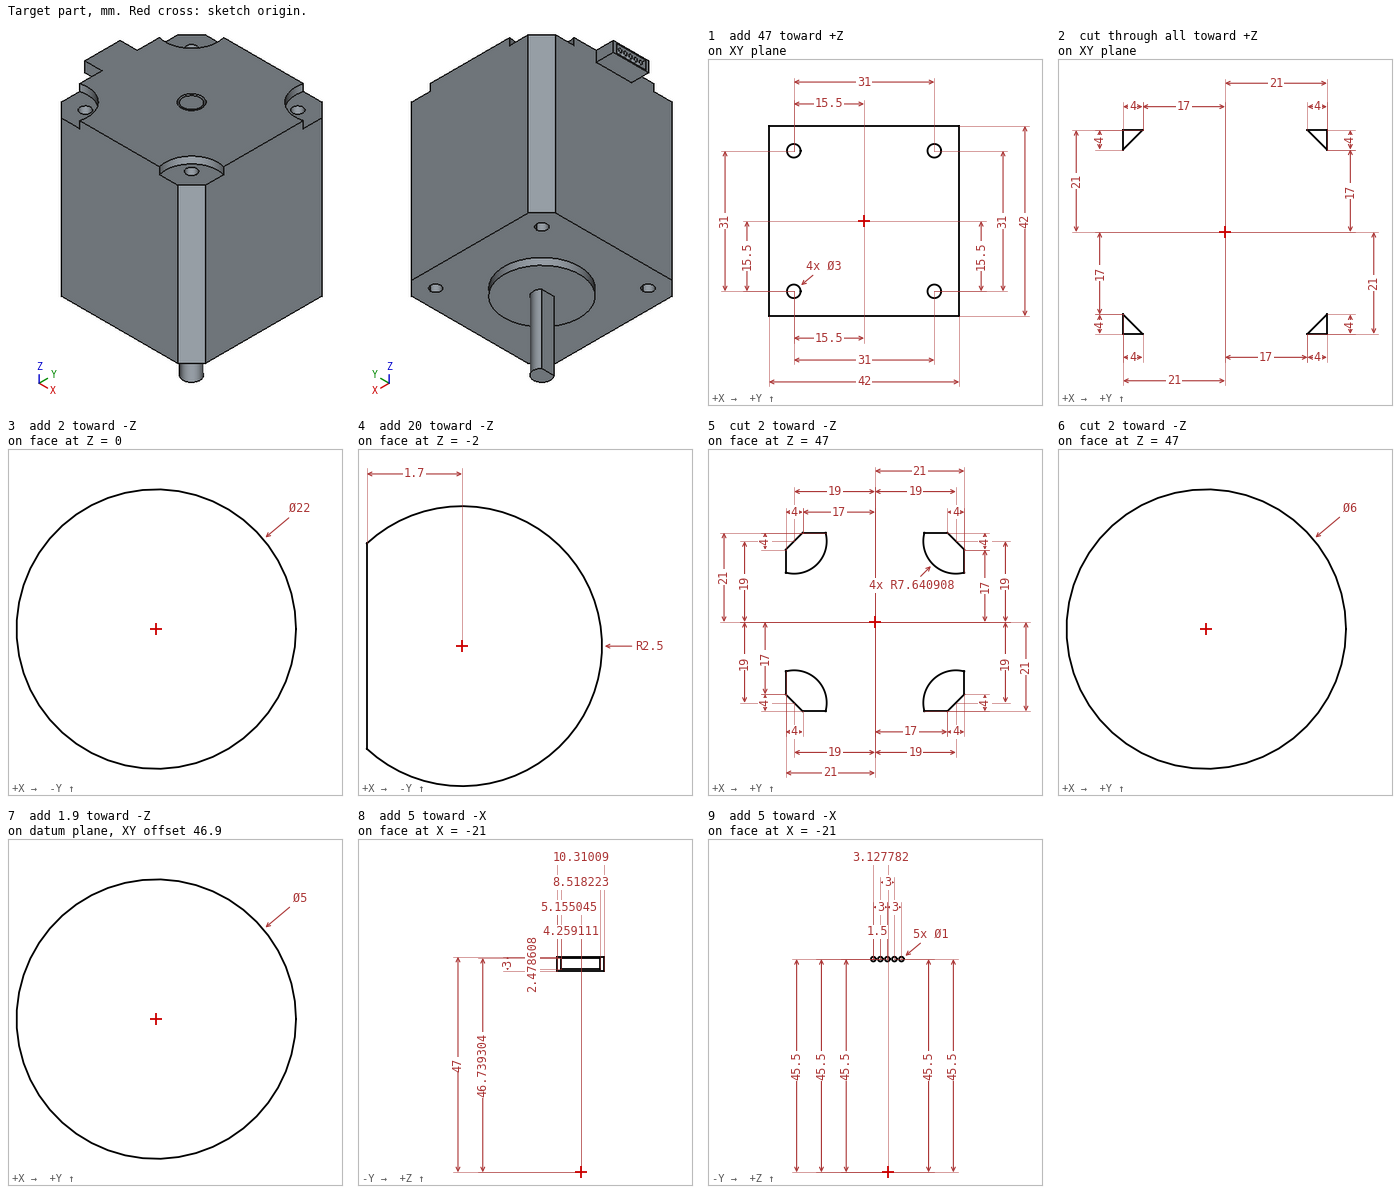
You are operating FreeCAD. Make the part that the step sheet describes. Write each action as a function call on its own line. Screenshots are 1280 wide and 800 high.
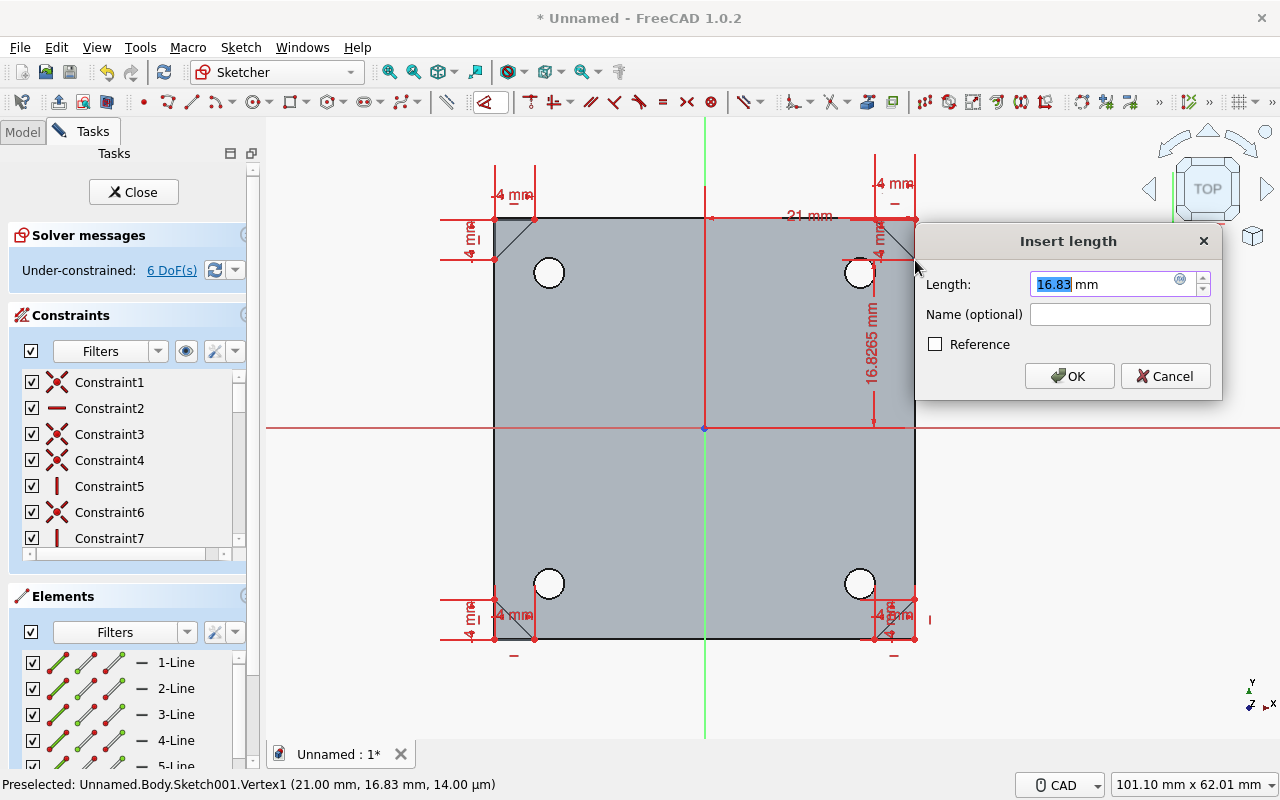
text(17)
key(Return)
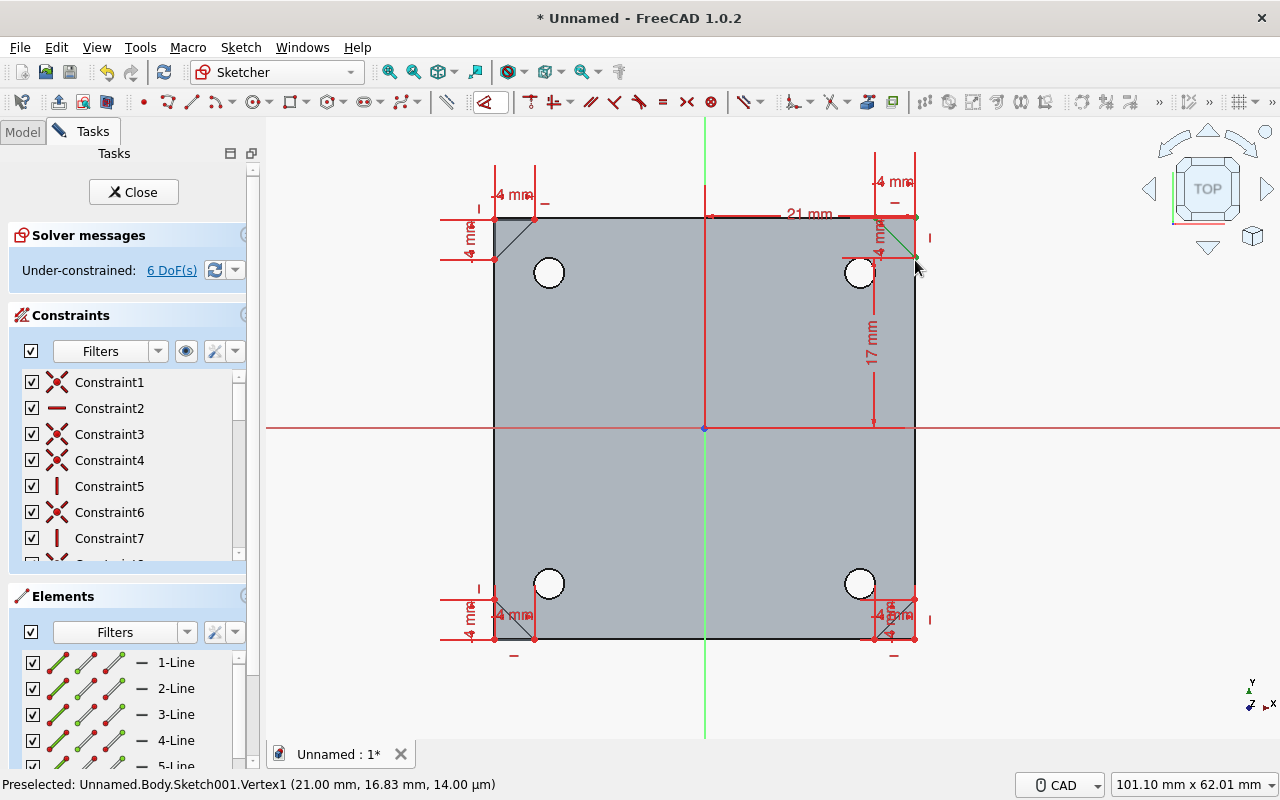
click(535, 220)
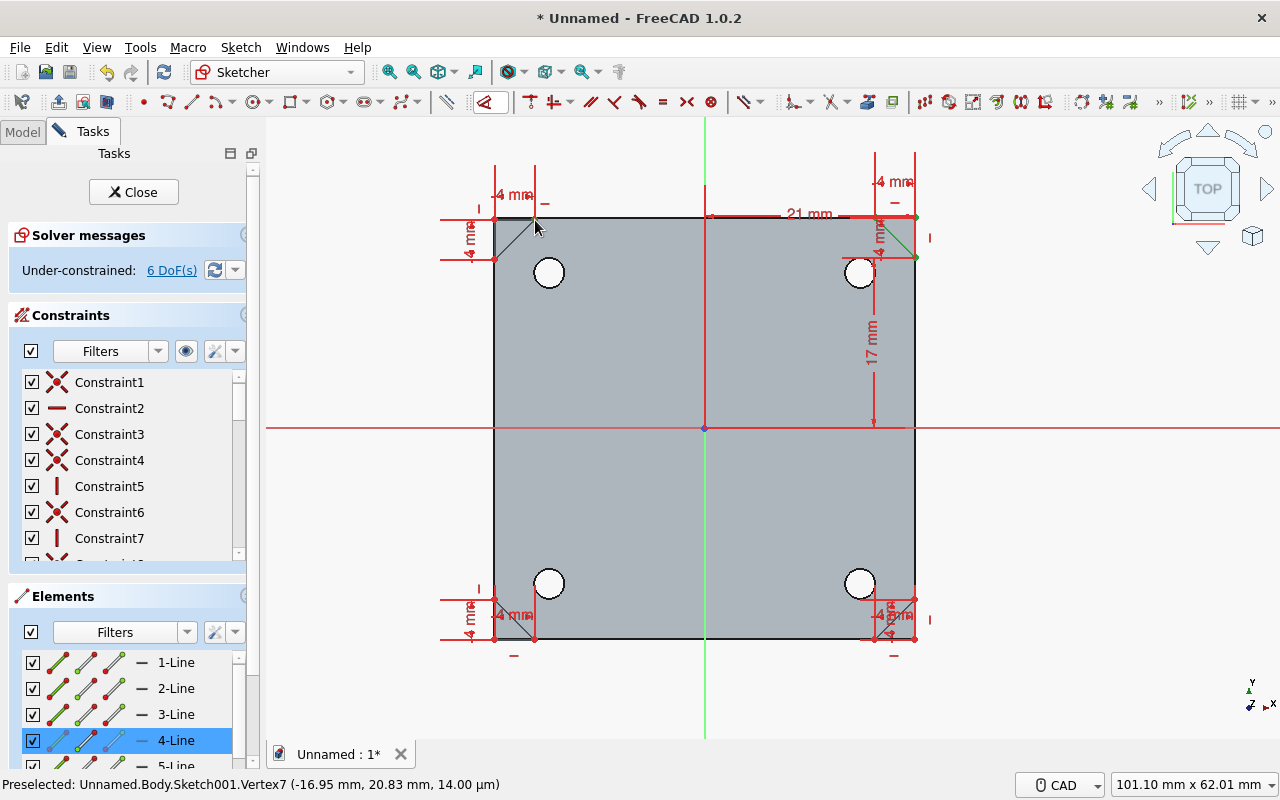
click(502, 102)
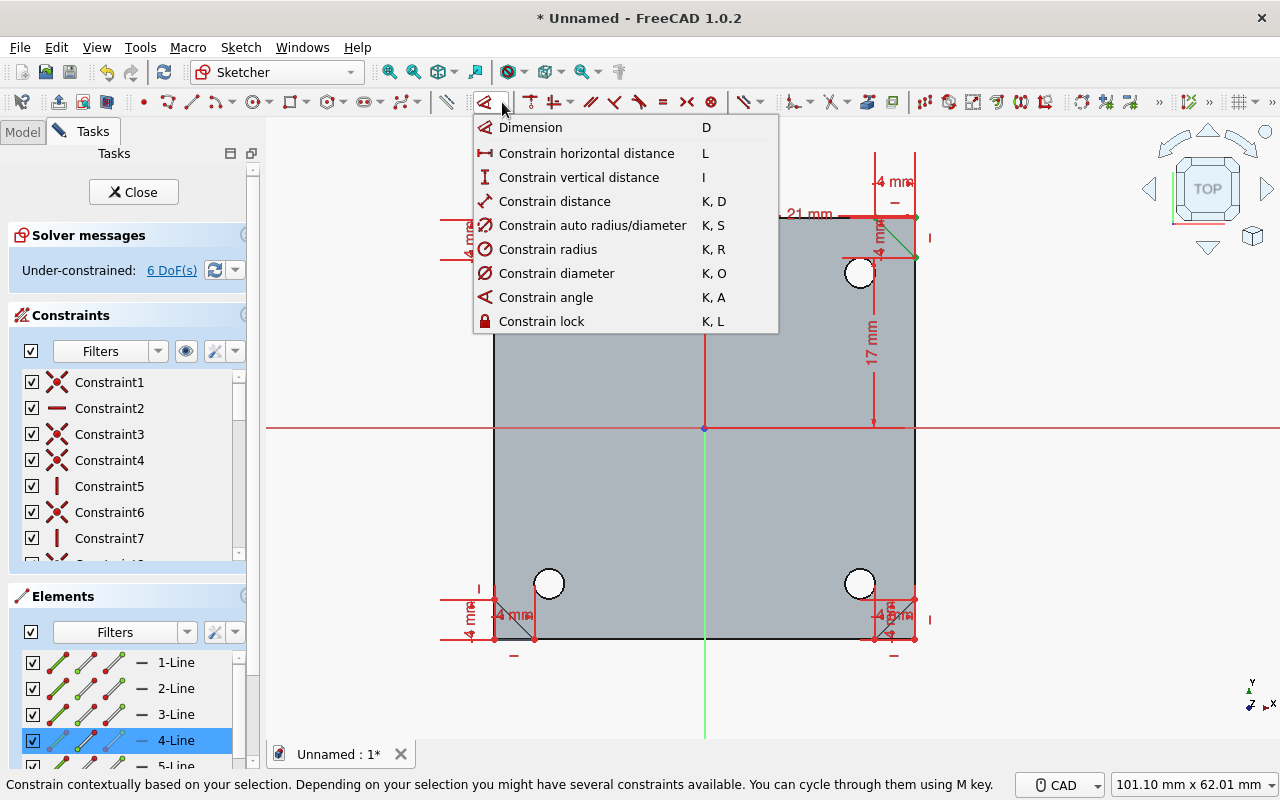
click(626, 153)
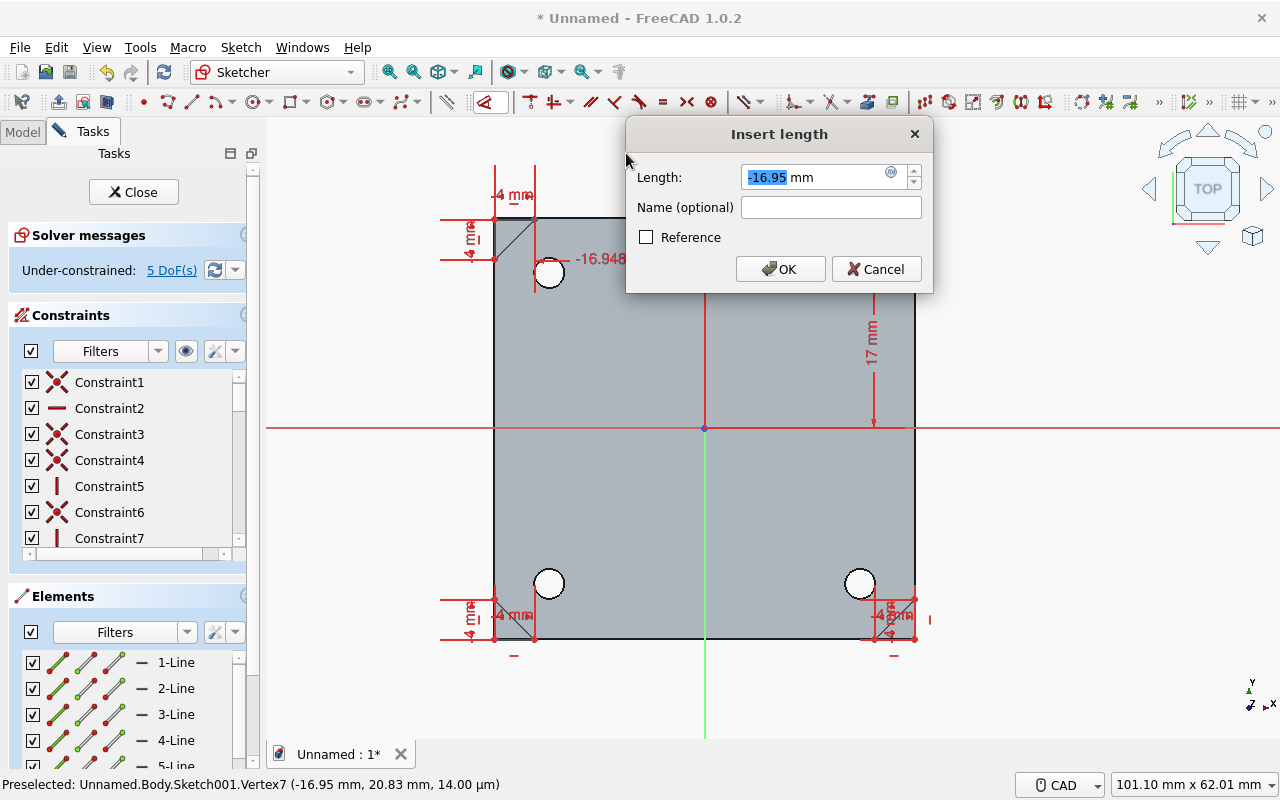
text(-17)
key(Return)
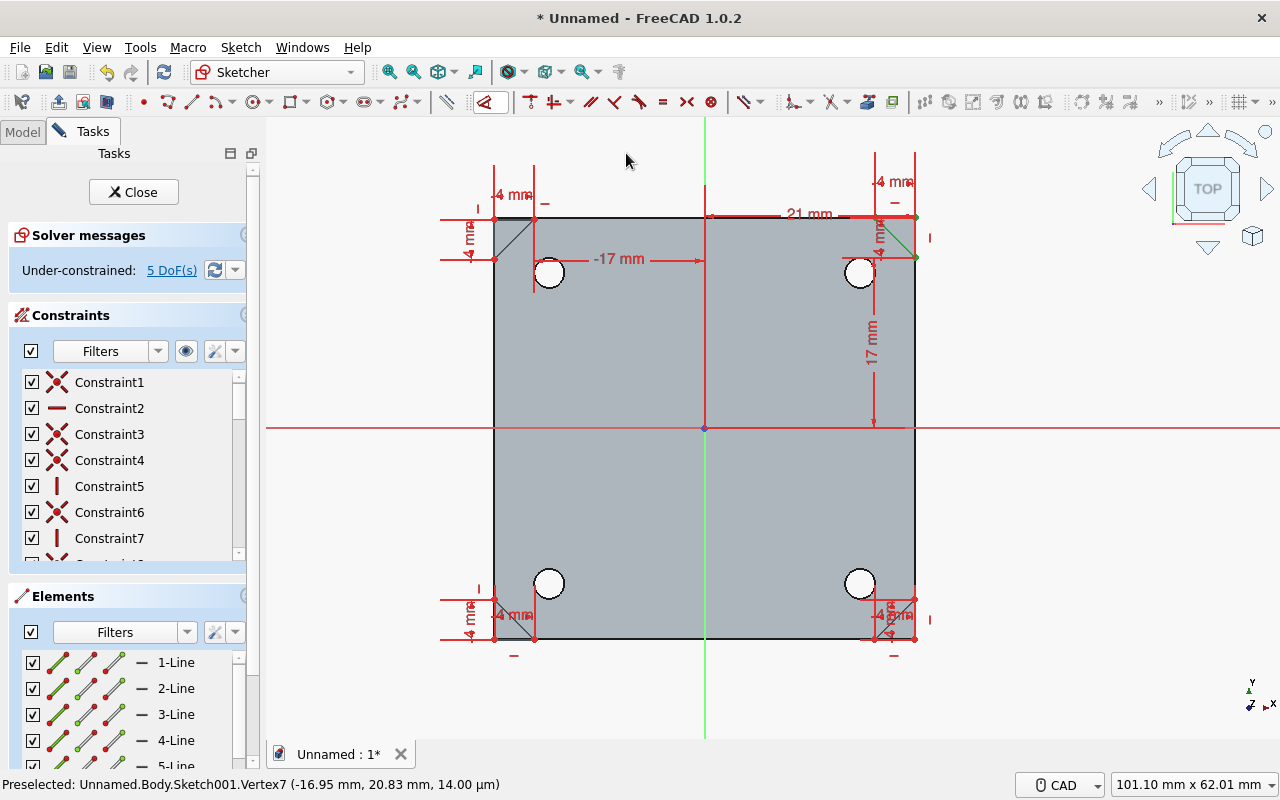
click(534, 220)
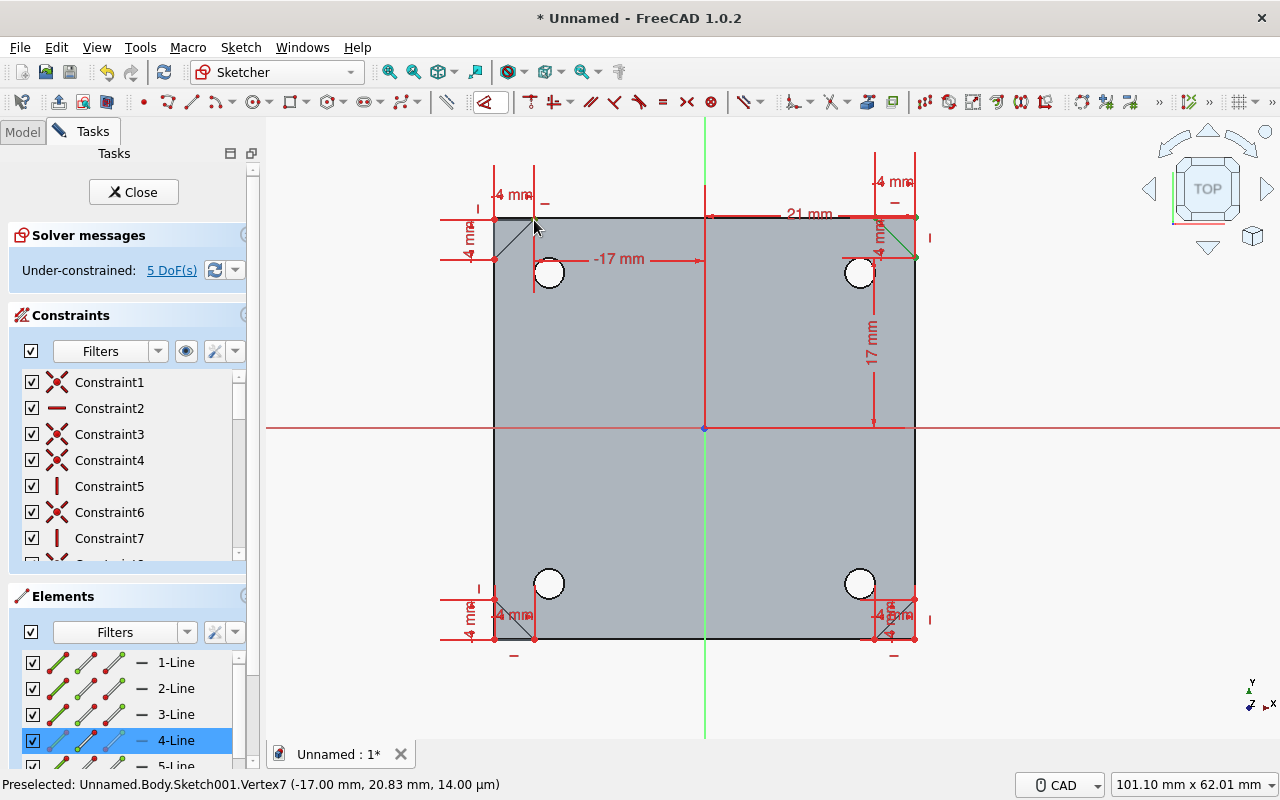
key(i)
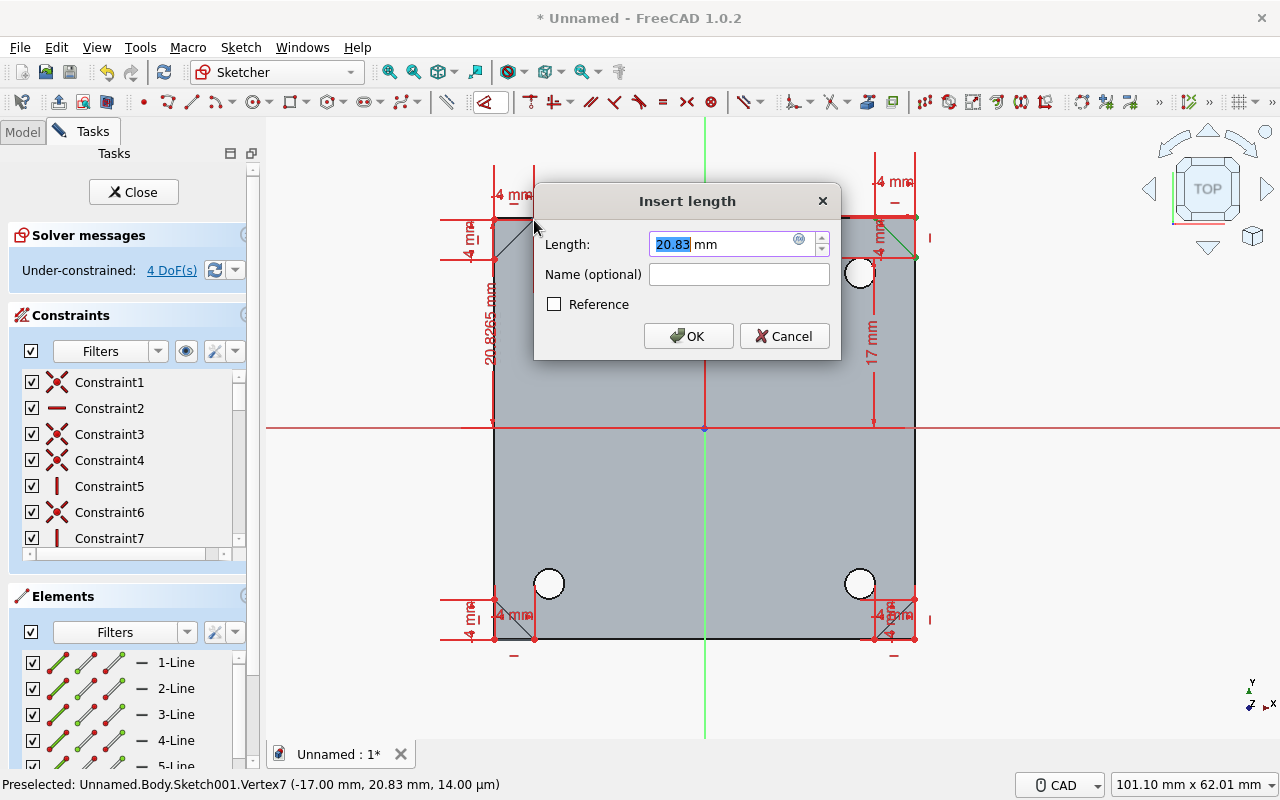
text(21)
key(Return)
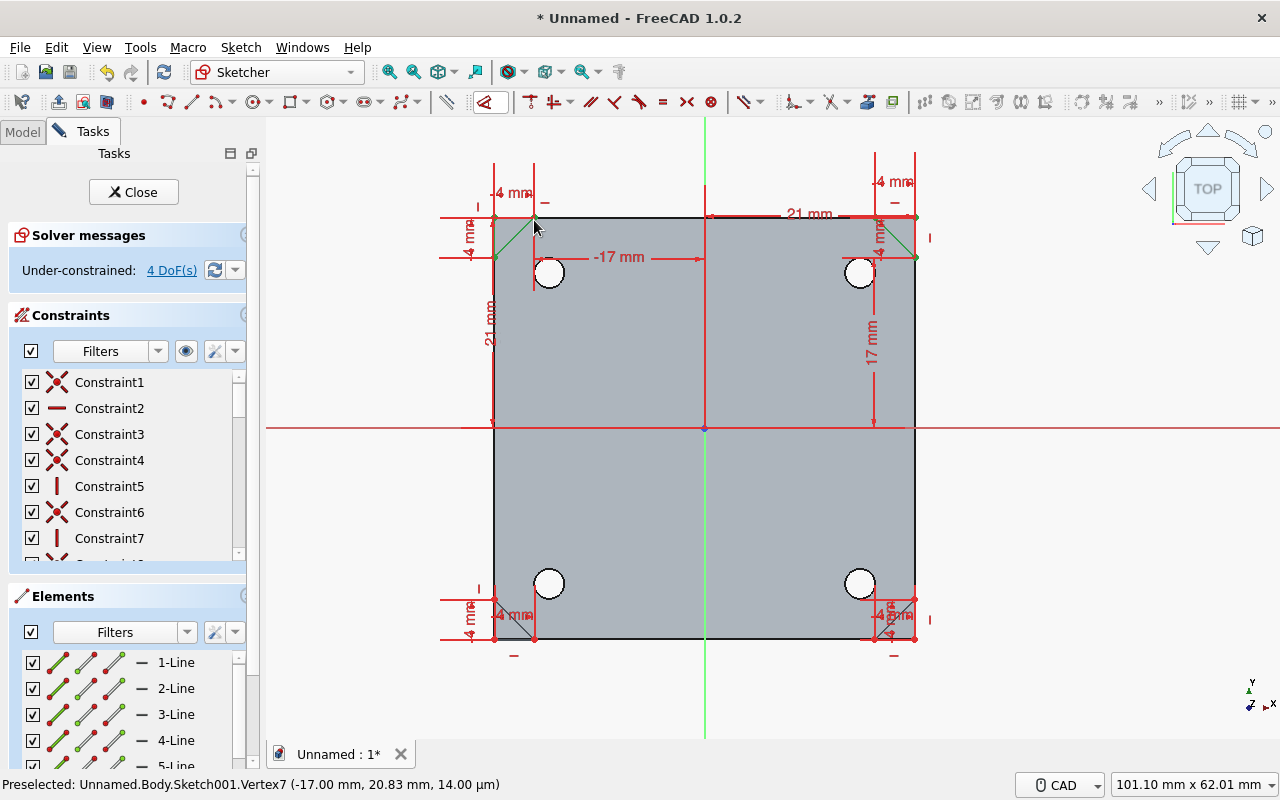
click(495, 600)